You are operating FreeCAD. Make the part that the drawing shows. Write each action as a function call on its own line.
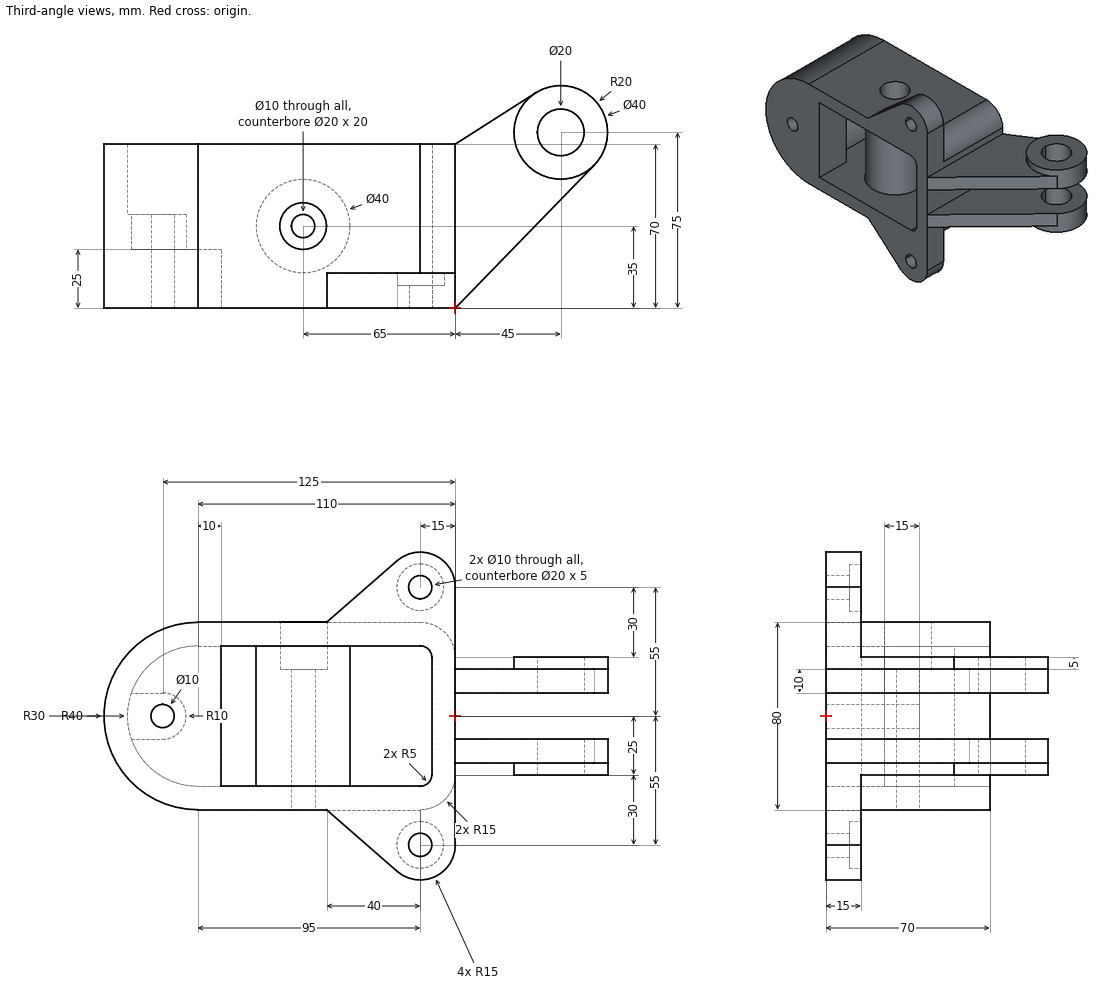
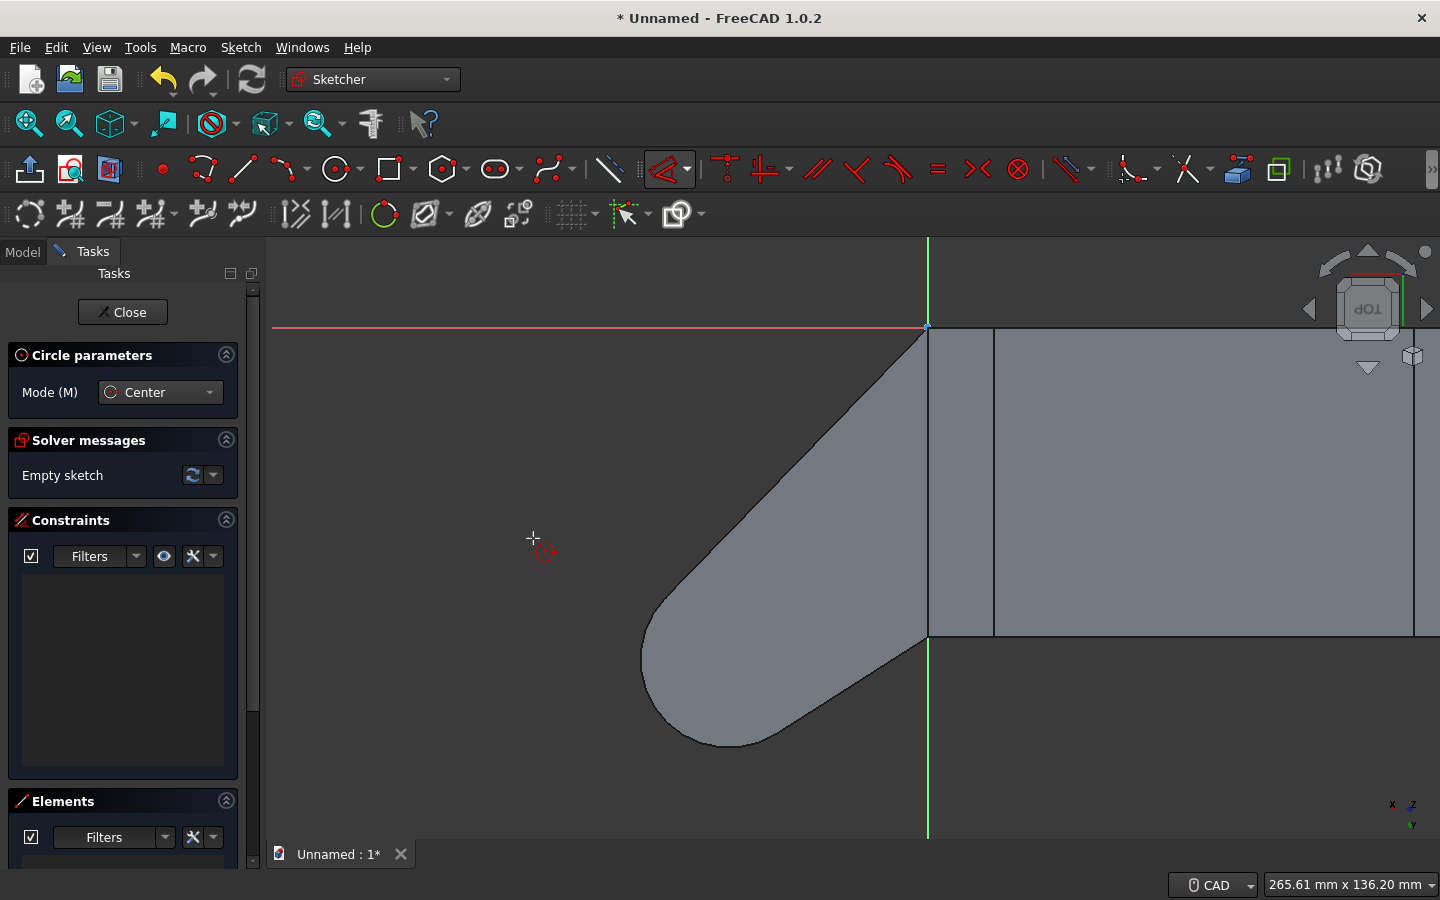
click(729, 659)
move(791, 597)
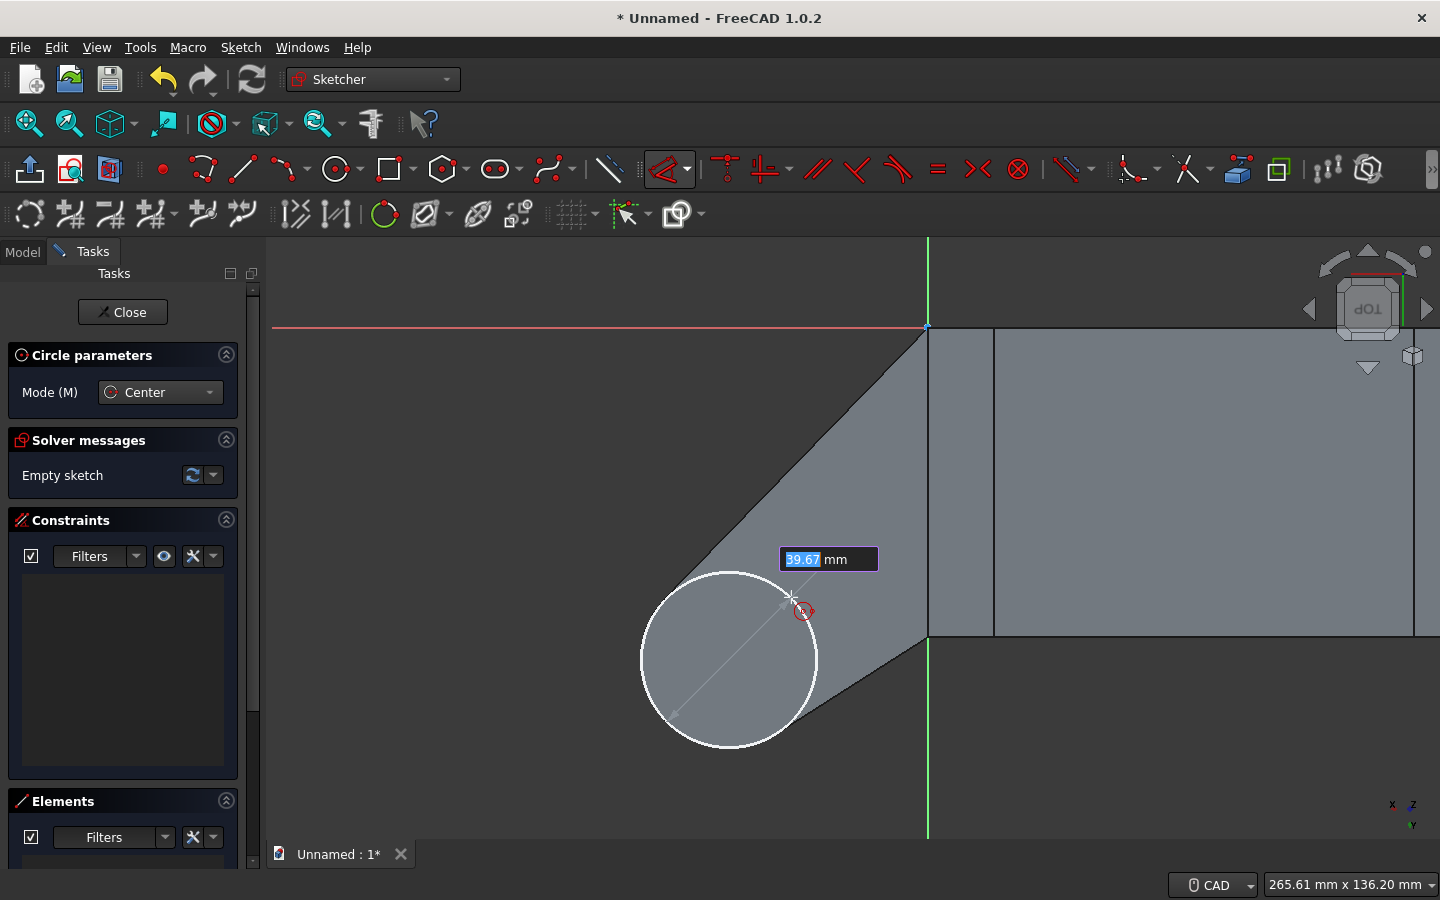
text(40)
key(Return)
key(Escape)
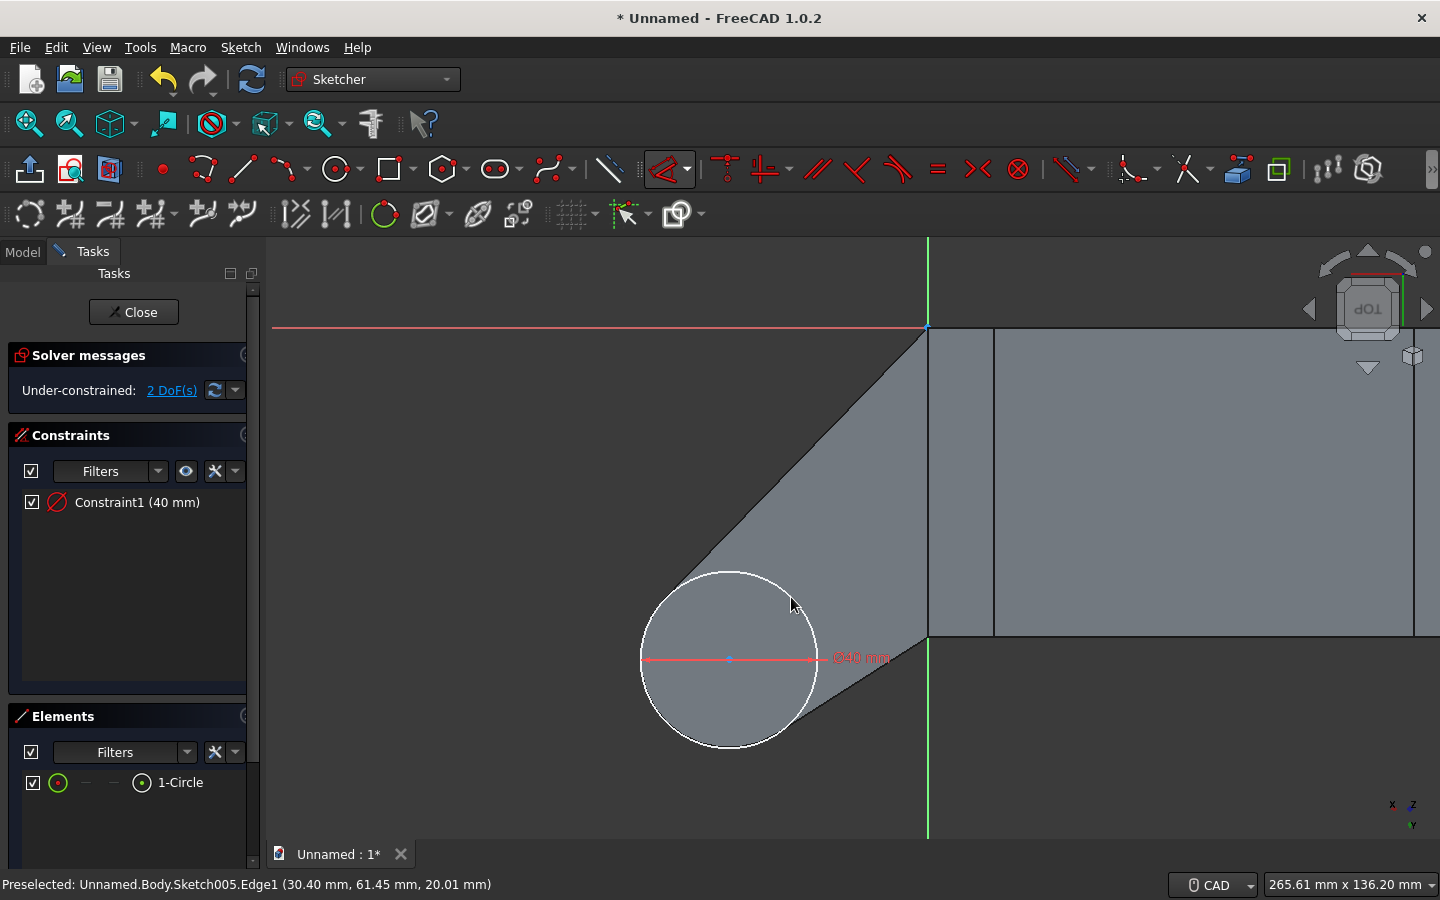
click(729, 660)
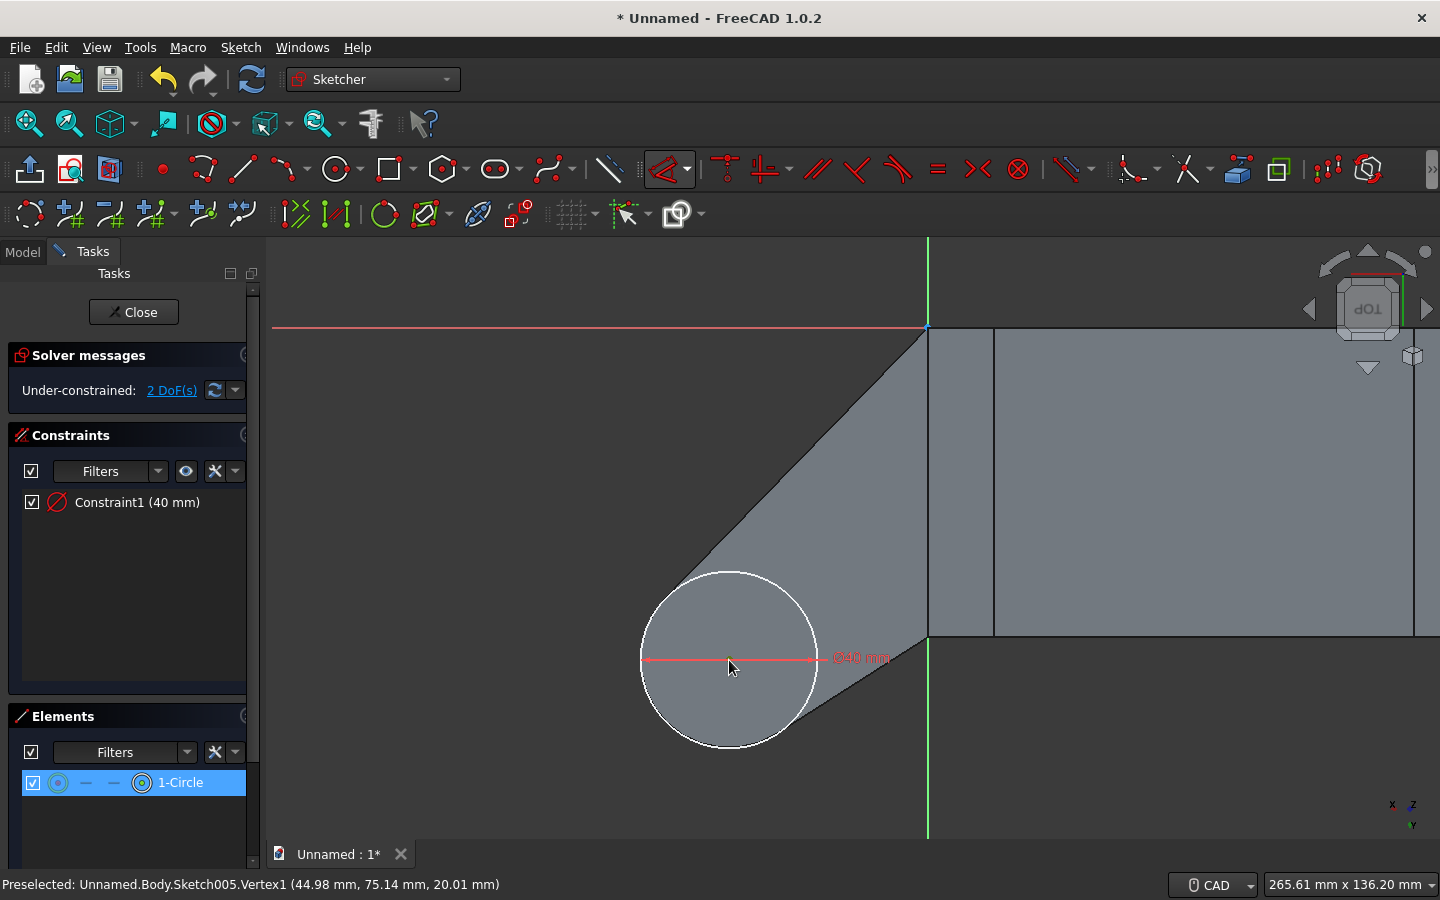
key(l)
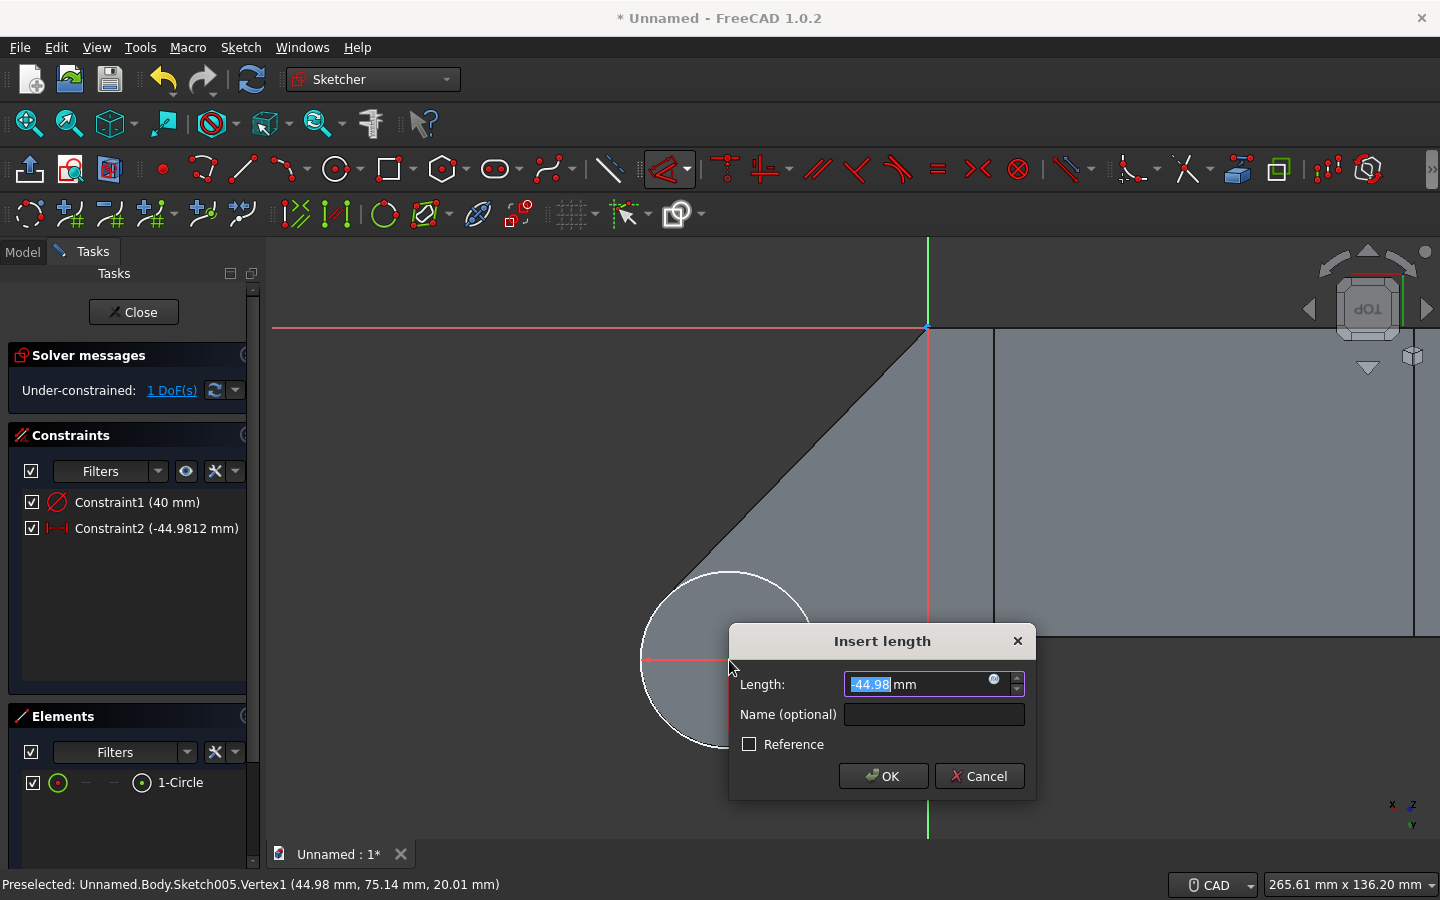
text(-45)
key(Return)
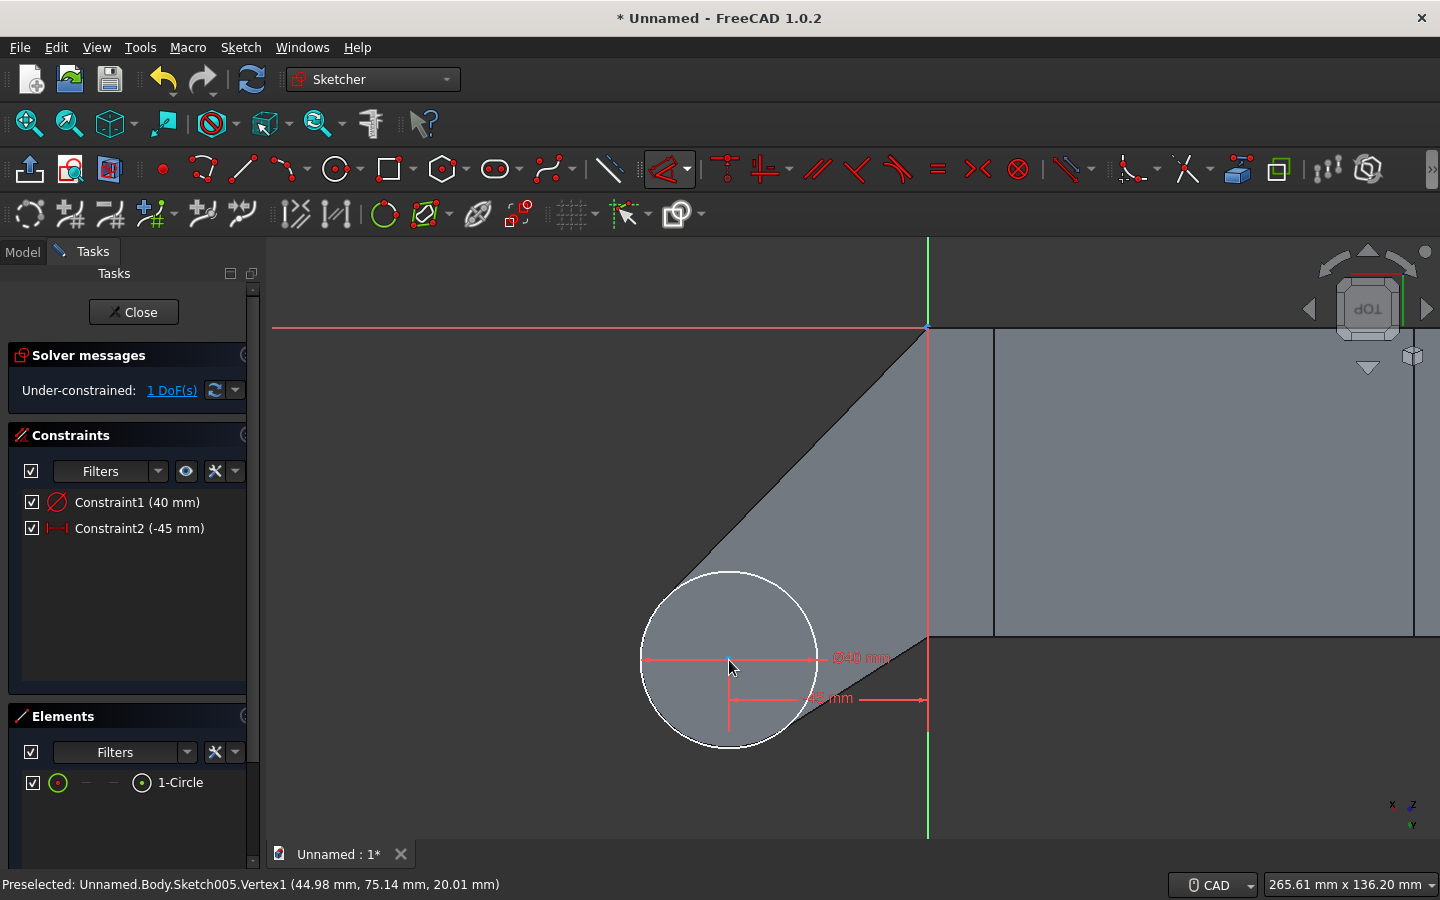
click(729, 660)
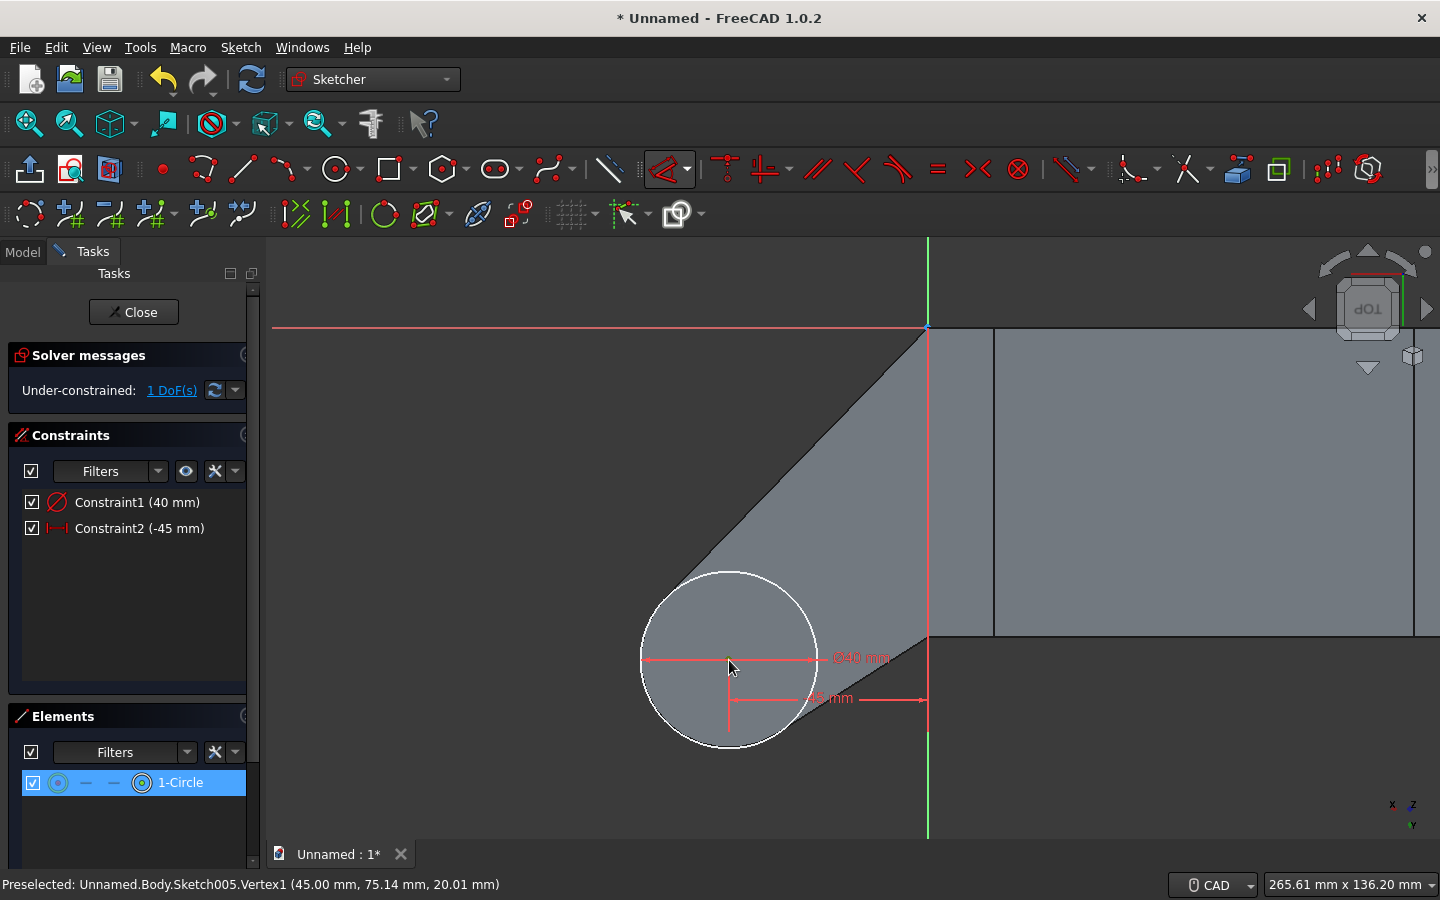
key(i)